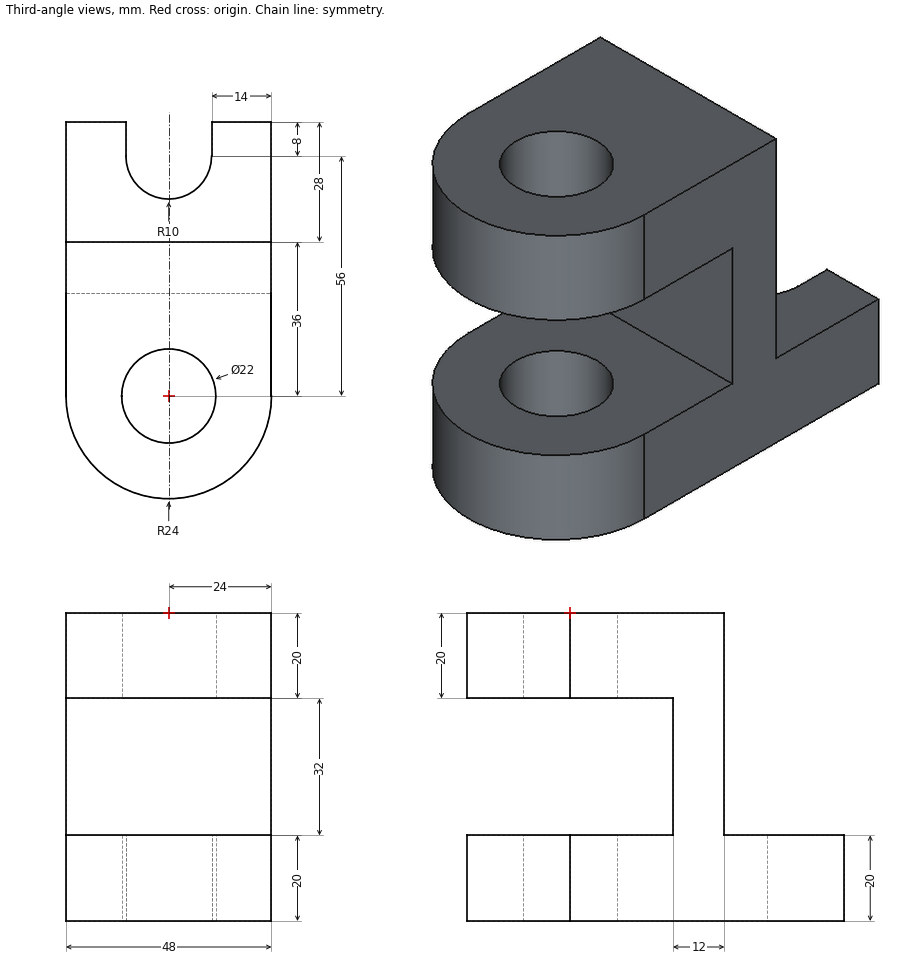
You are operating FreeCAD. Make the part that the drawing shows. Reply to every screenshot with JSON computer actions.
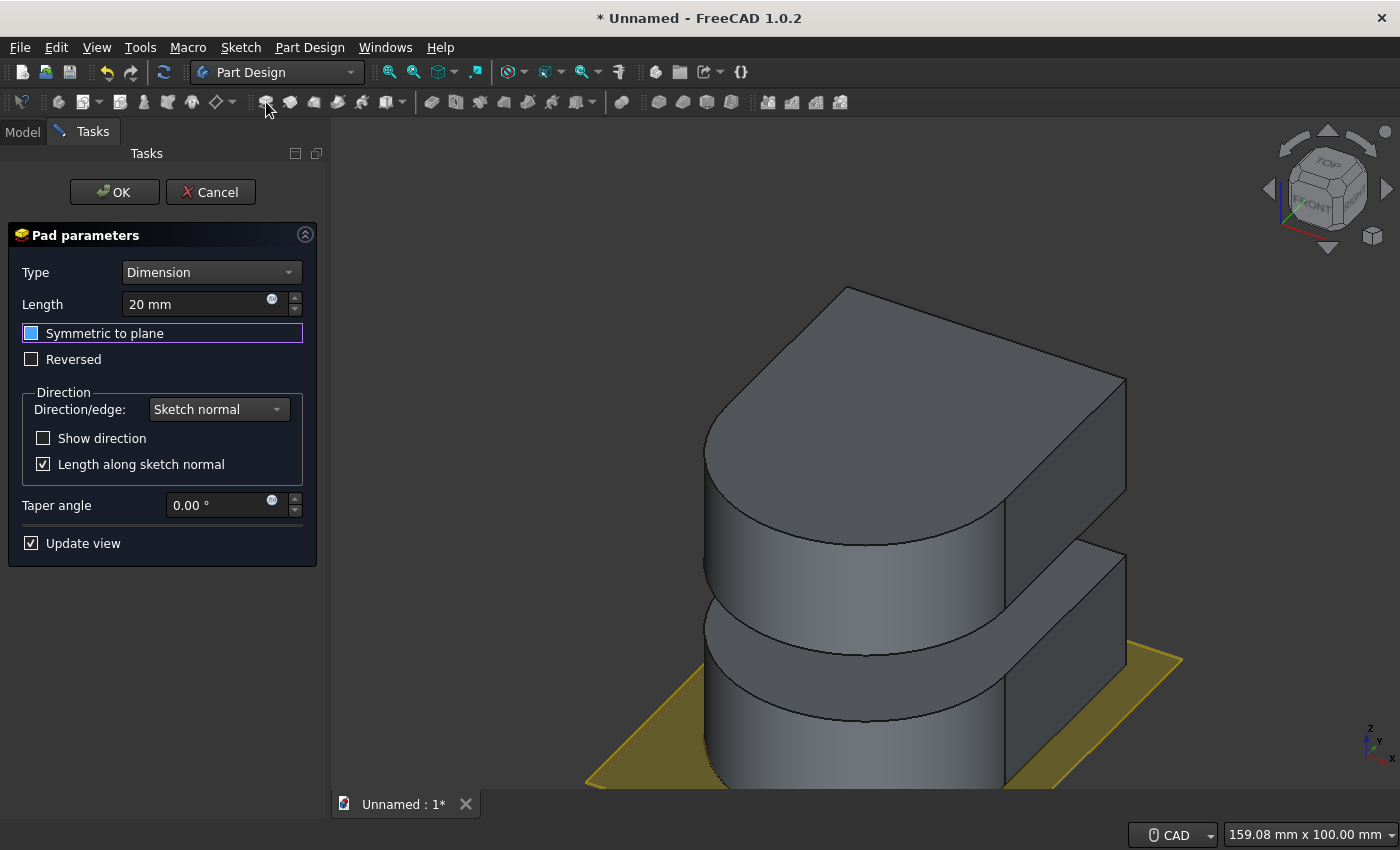
{"action": "left_click", "coordinate": [30, 359]}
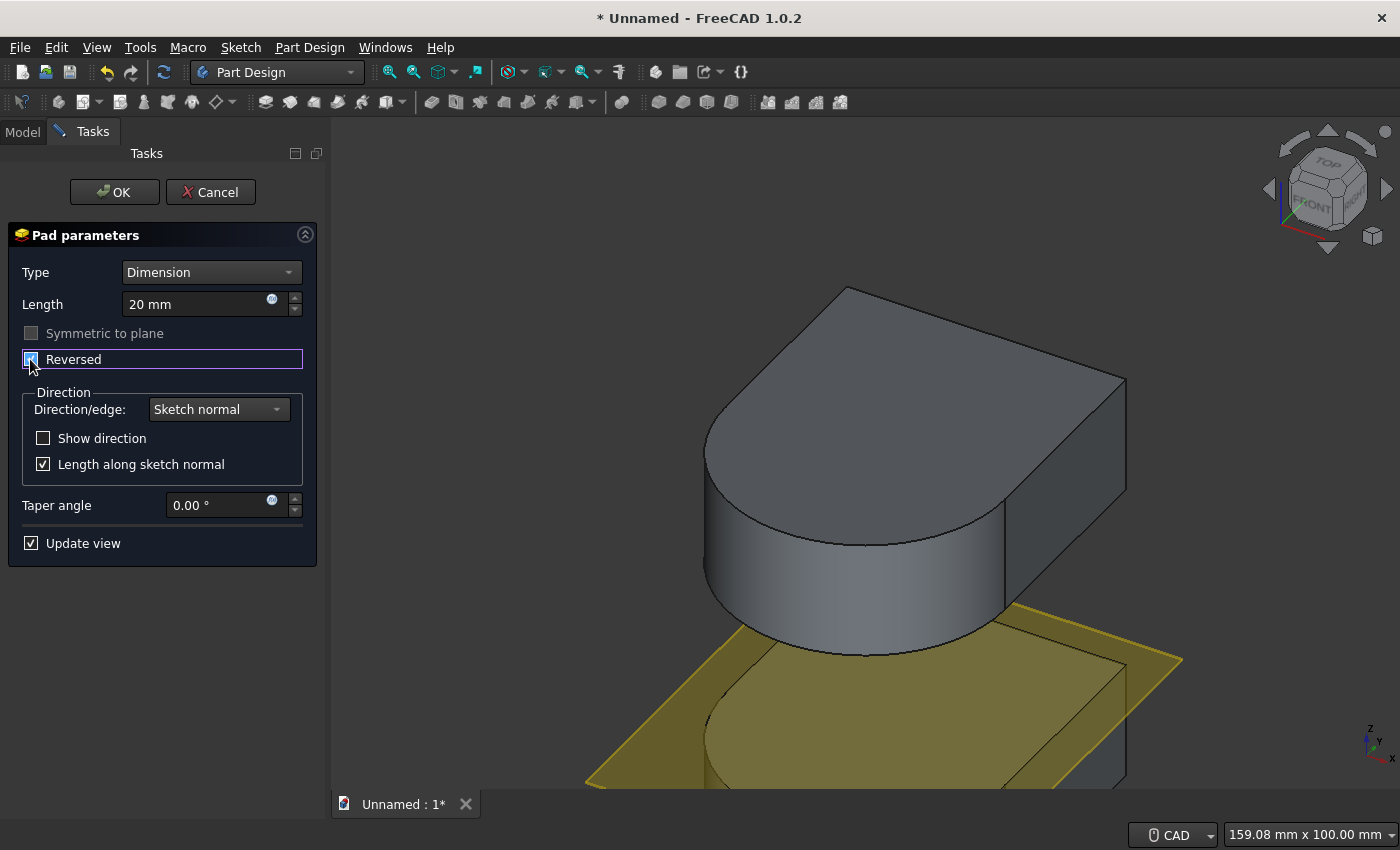
{"action": "left_click", "coordinate": [115, 192]}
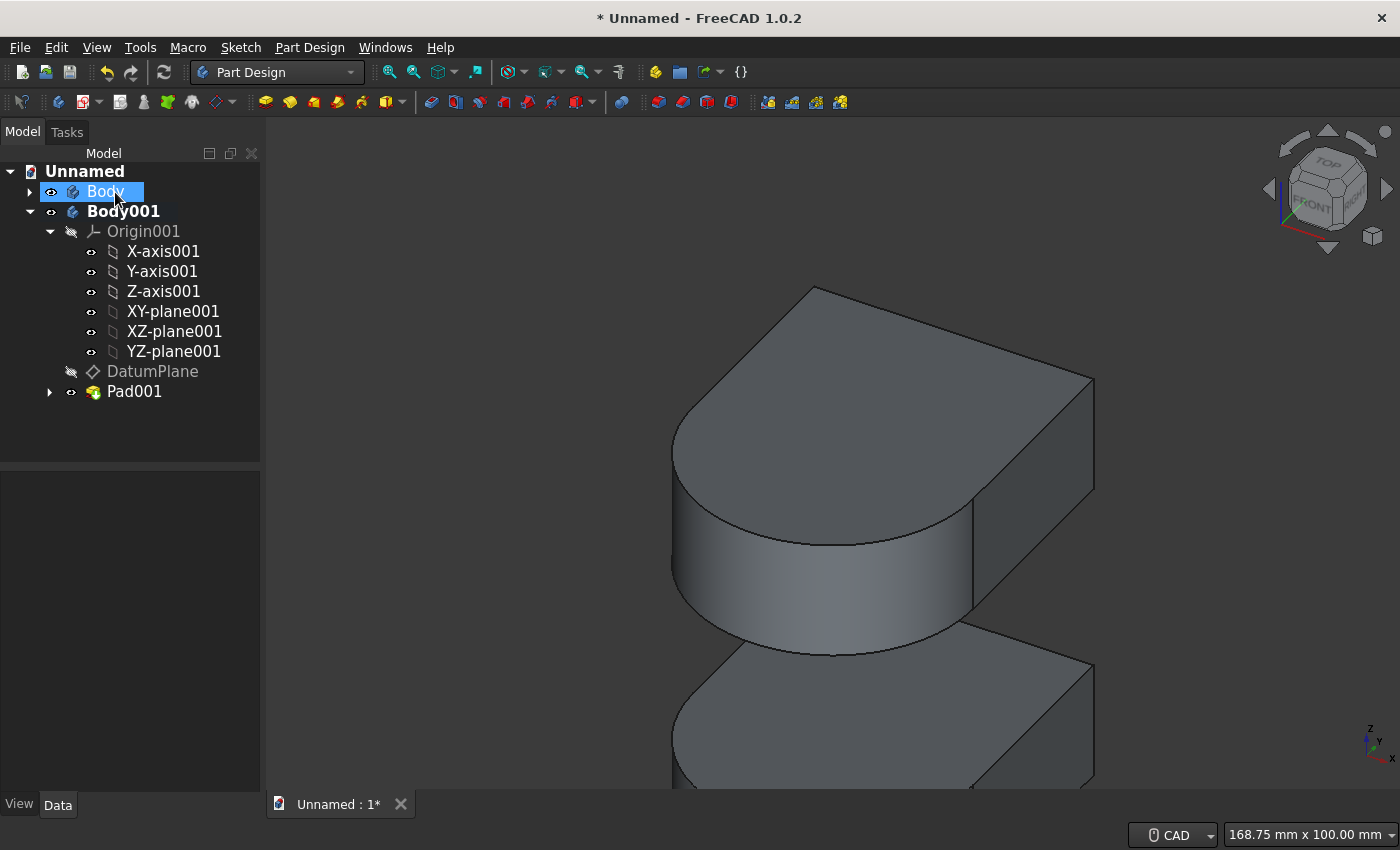
{"action": "left_click", "coordinate": [390, 72]}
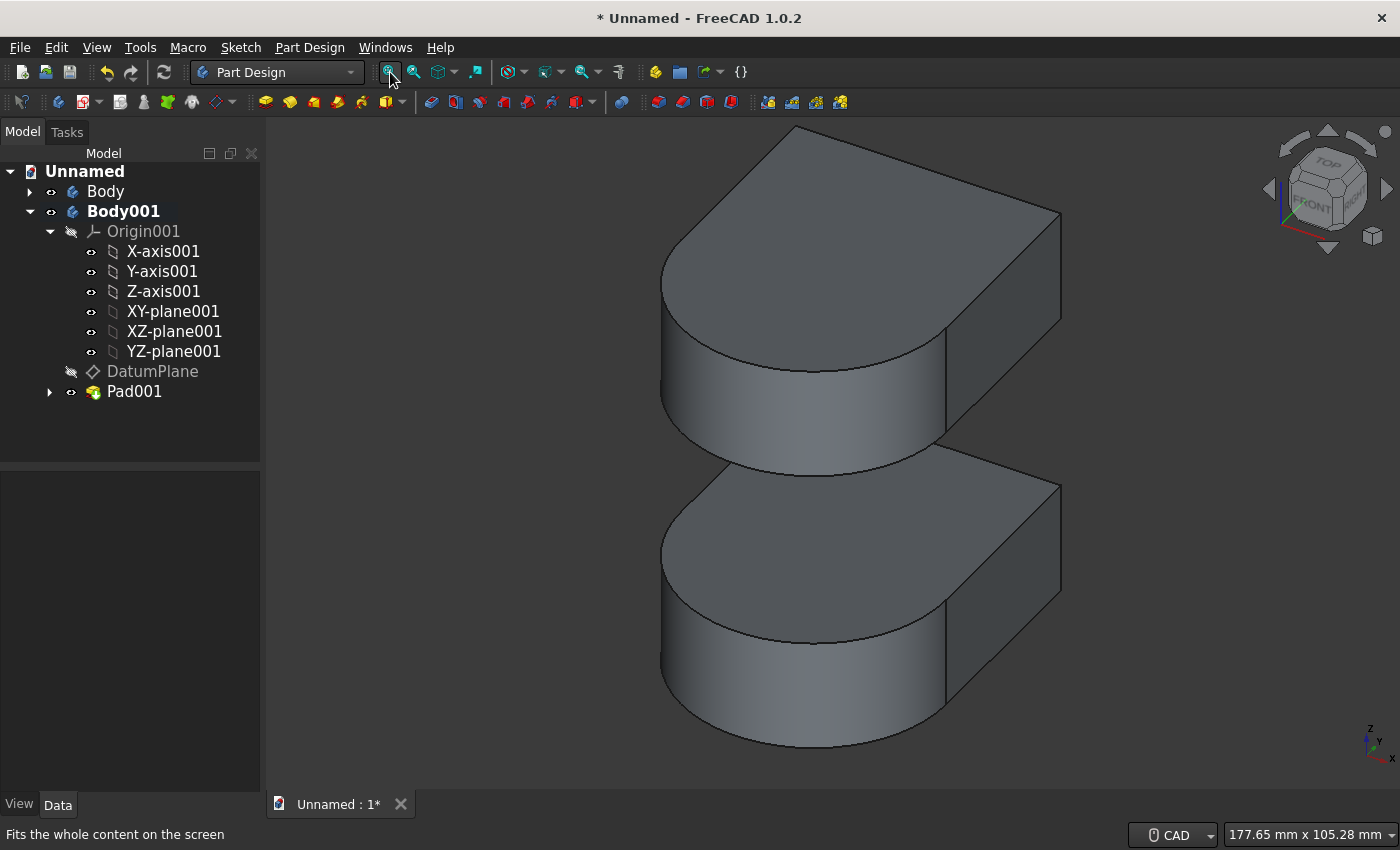
{"action": "double_click", "coordinate": [96, 192]}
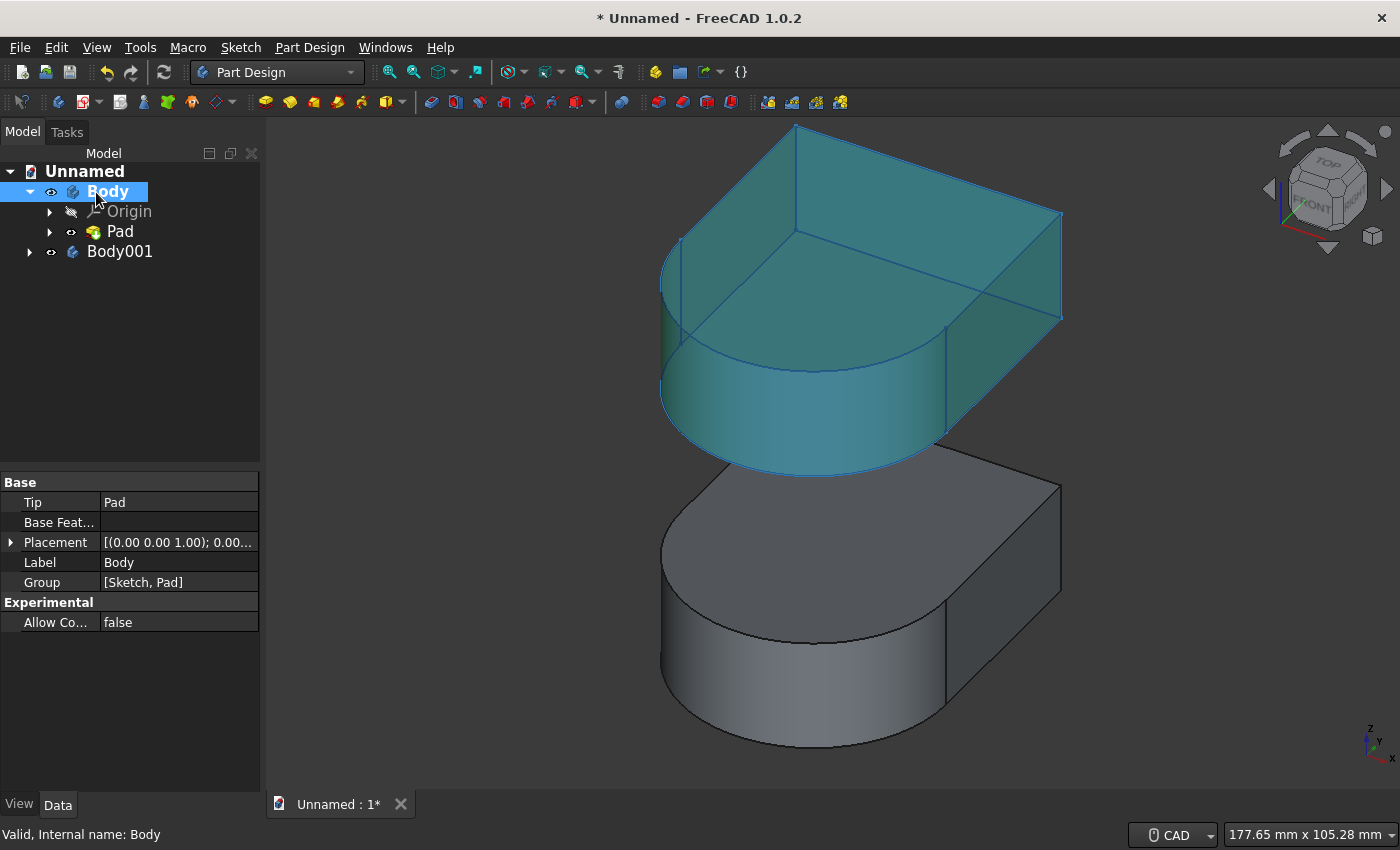
{"action": "left_click", "coordinate": [96, 192]}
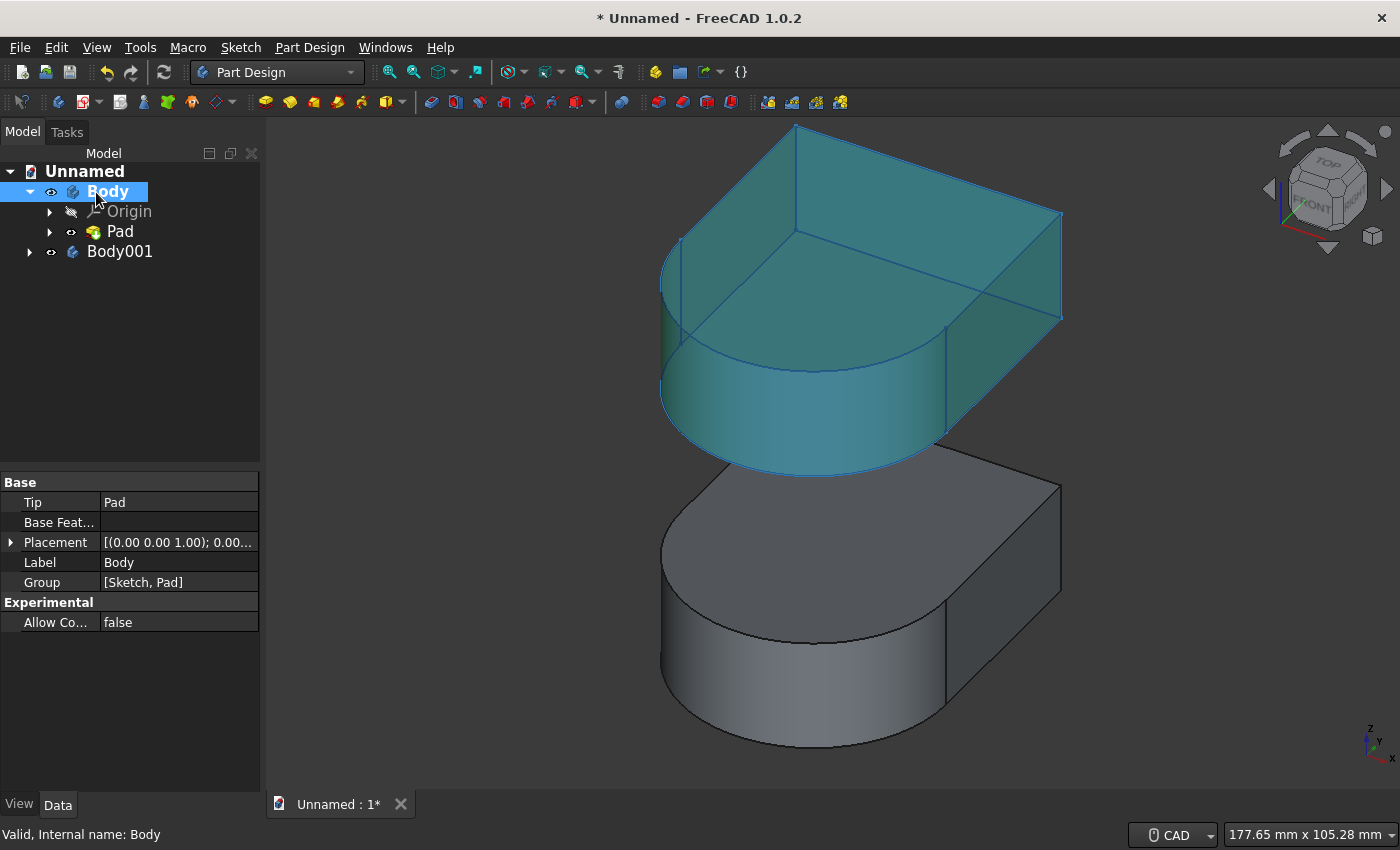
{"action": "left_click", "coordinate": [146, 622]}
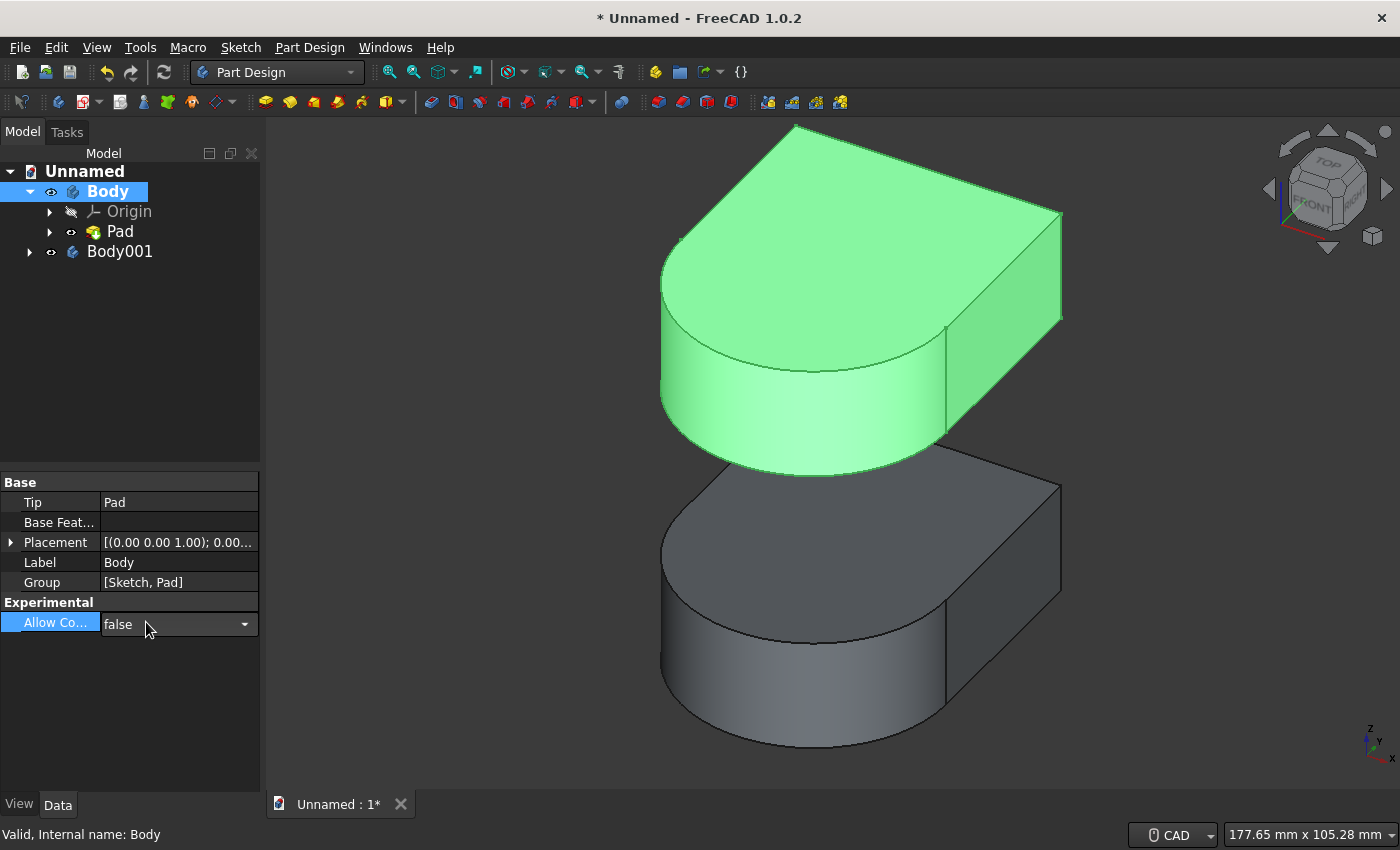
{"action": "left_click", "coordinate": [146, 622]}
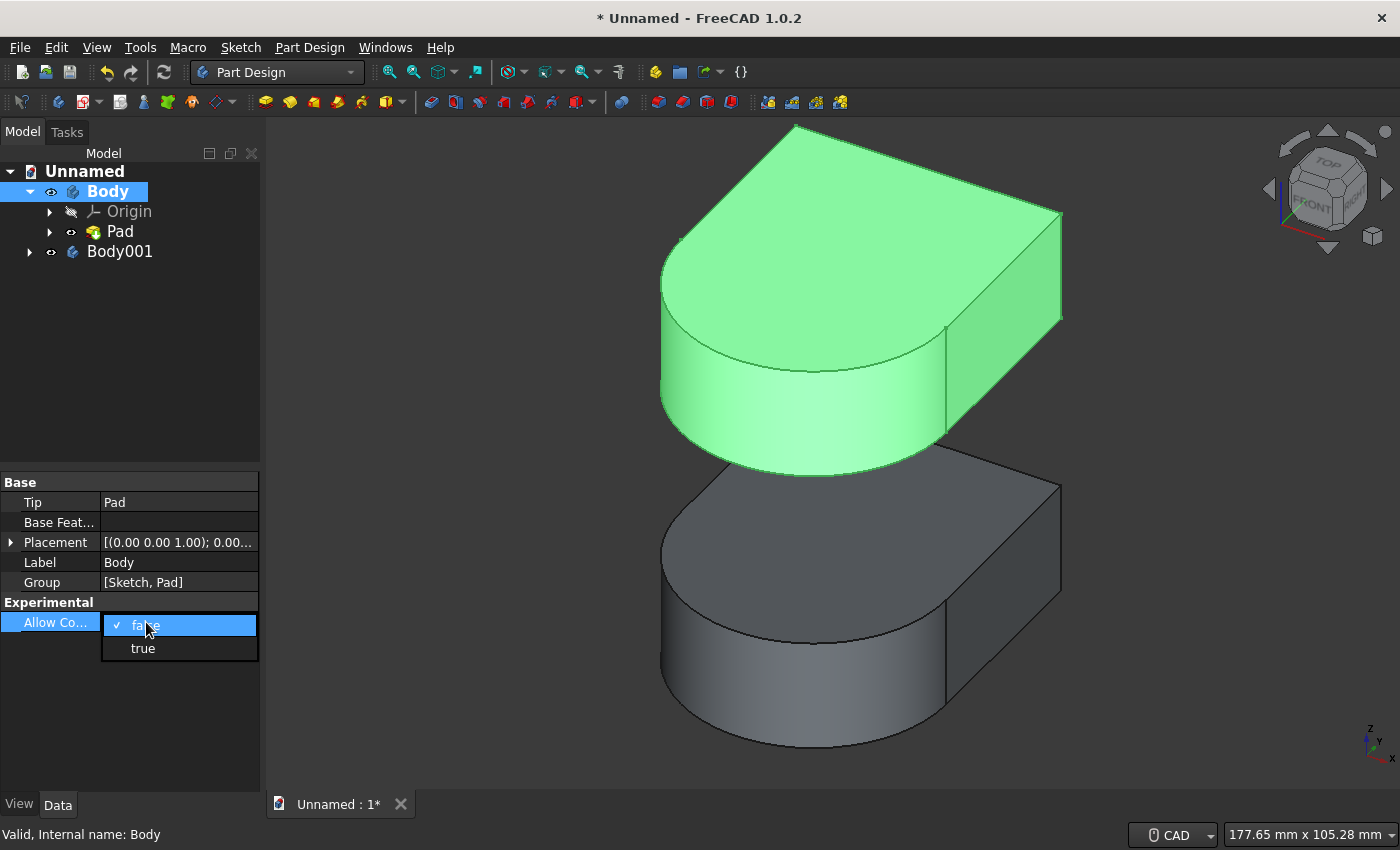
{"action": "left_click", "coordinate": [179, 648]}
{"action": "key", "text": "Return"}